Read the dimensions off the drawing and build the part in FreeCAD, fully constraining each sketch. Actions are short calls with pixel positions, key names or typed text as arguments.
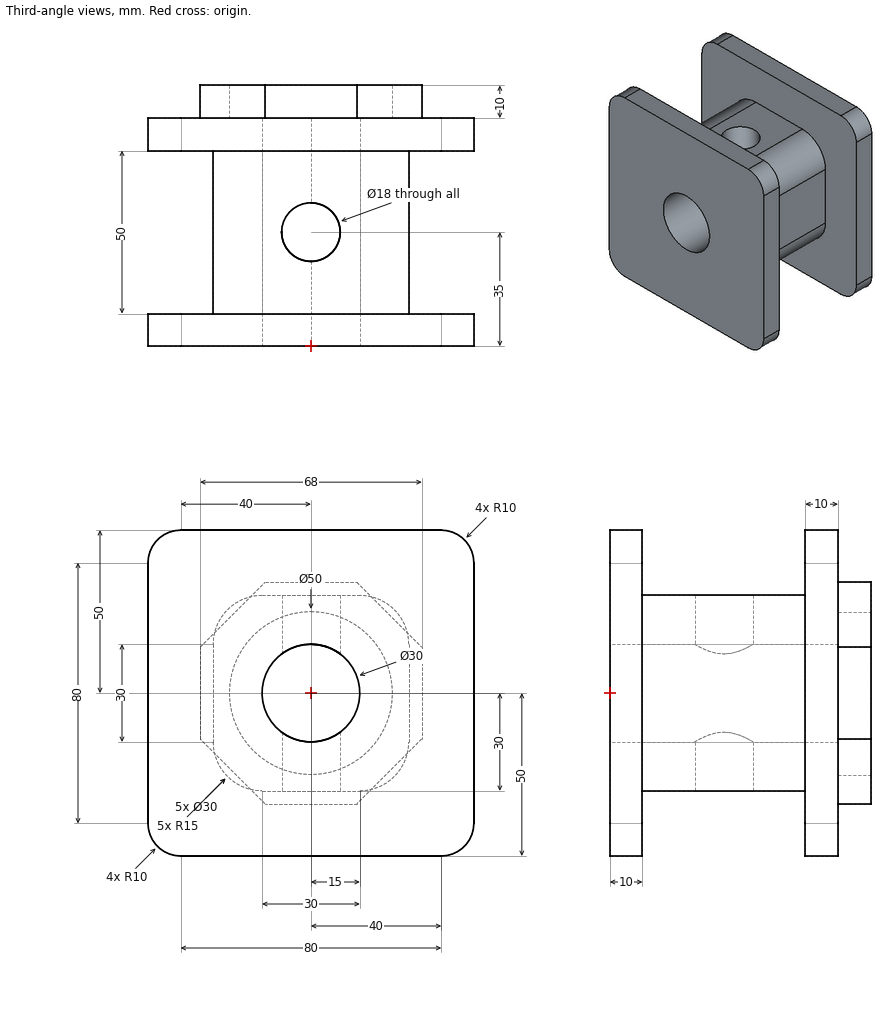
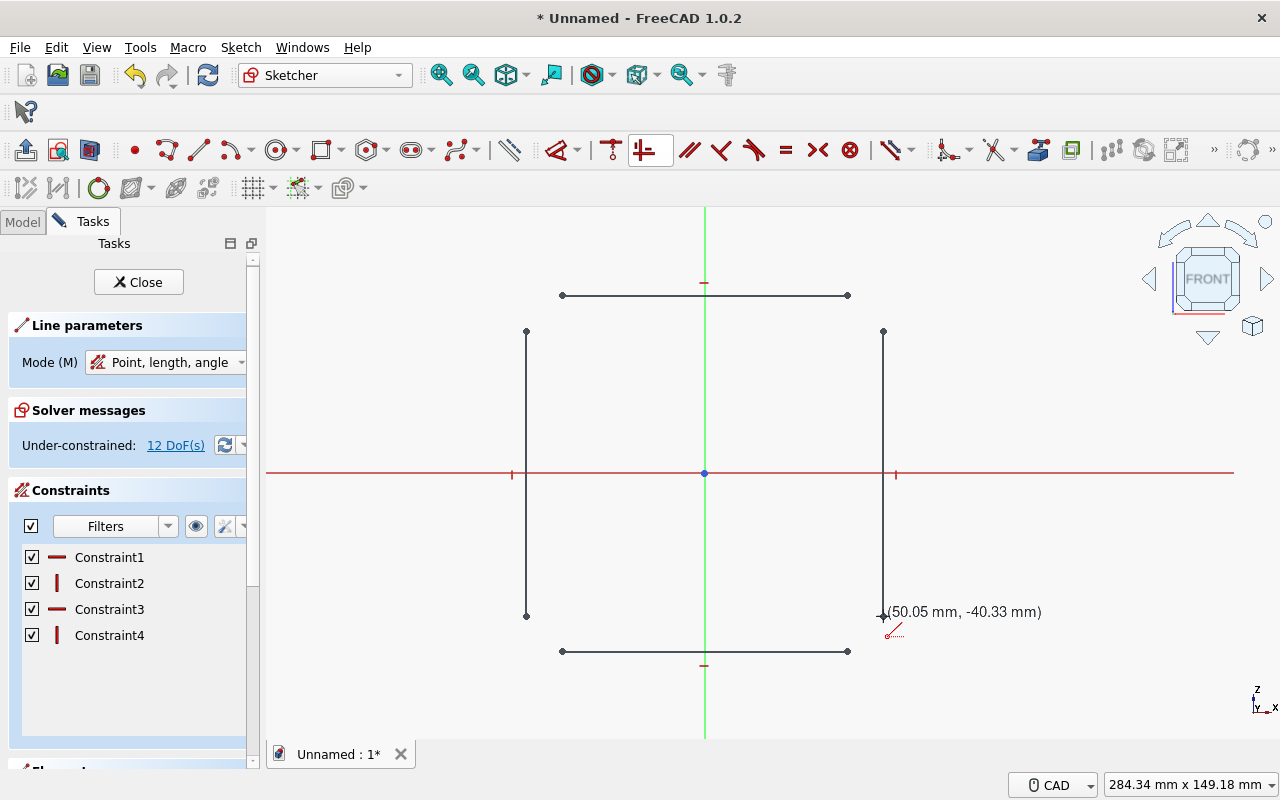
click(254, 150)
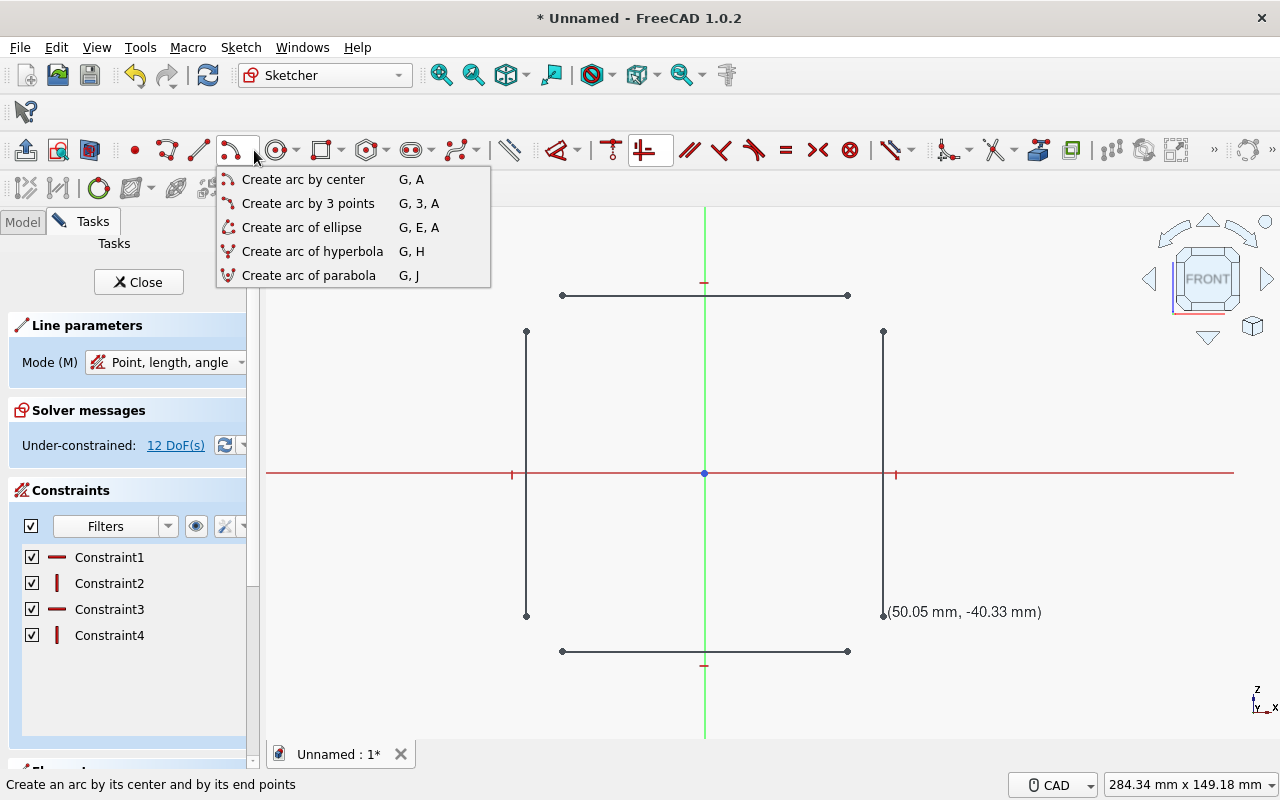
click(354, 203)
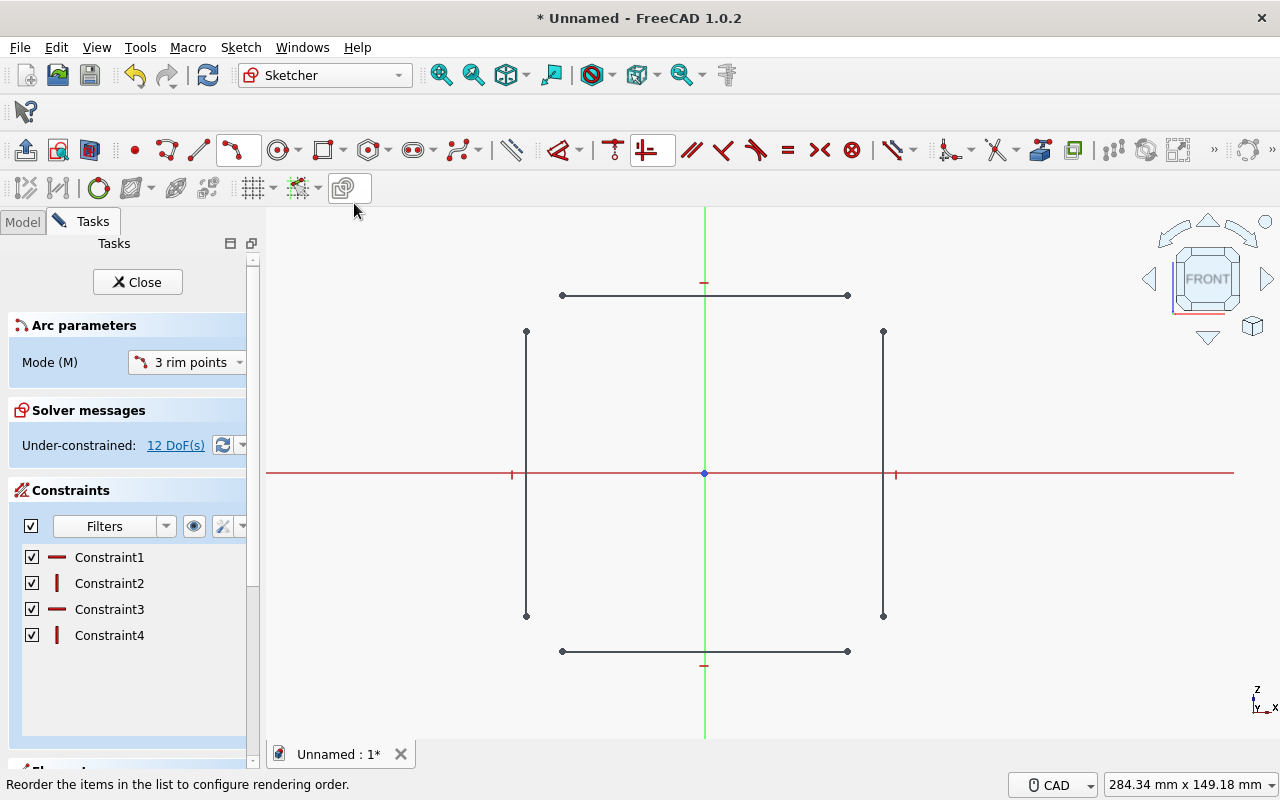
click(562, 652)
click(526, 617)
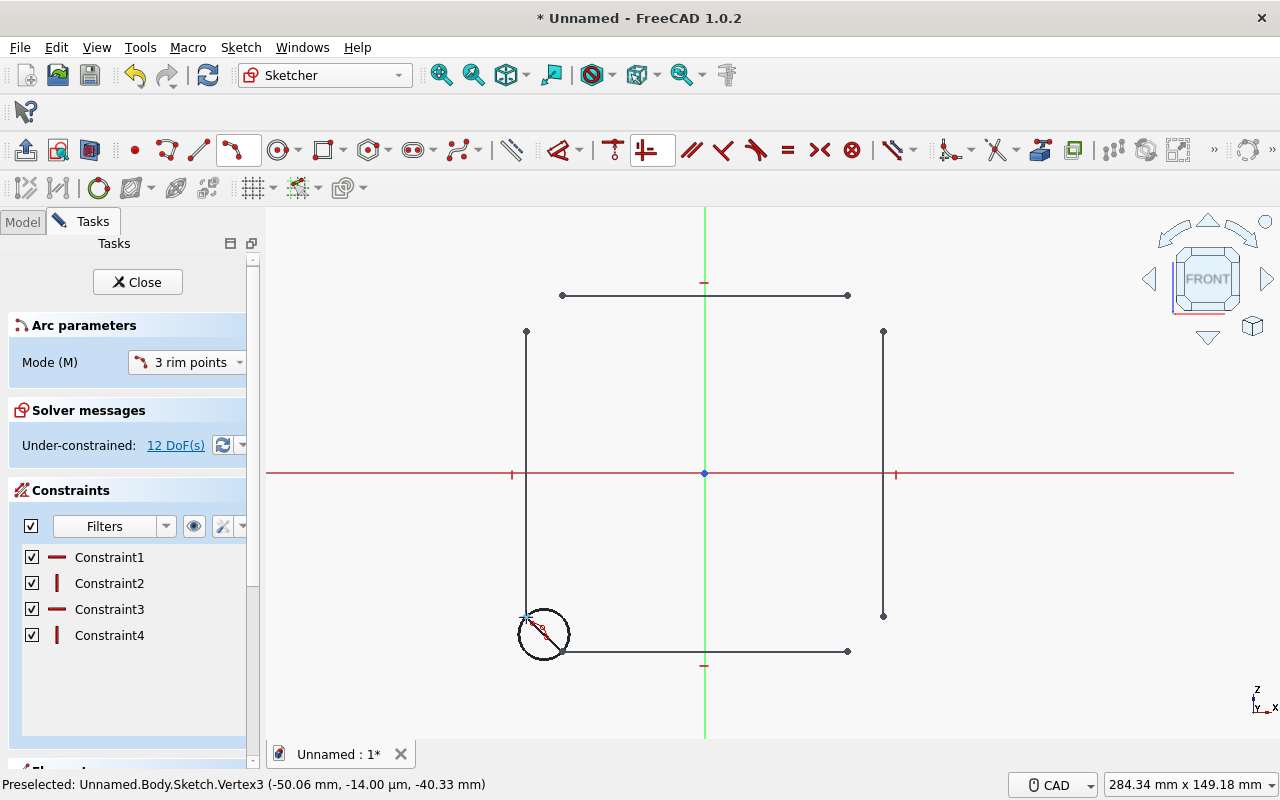
scroll(537, 641, up, 3)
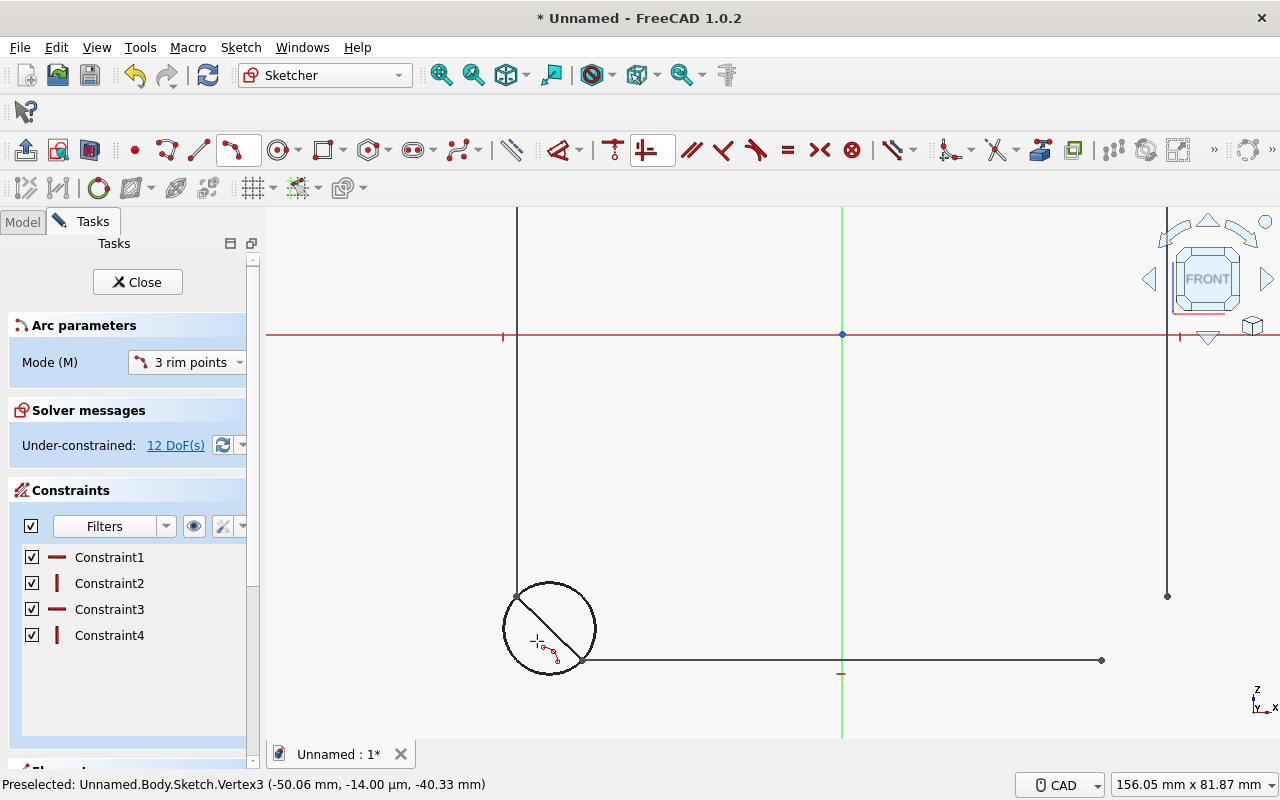
click(536, 640)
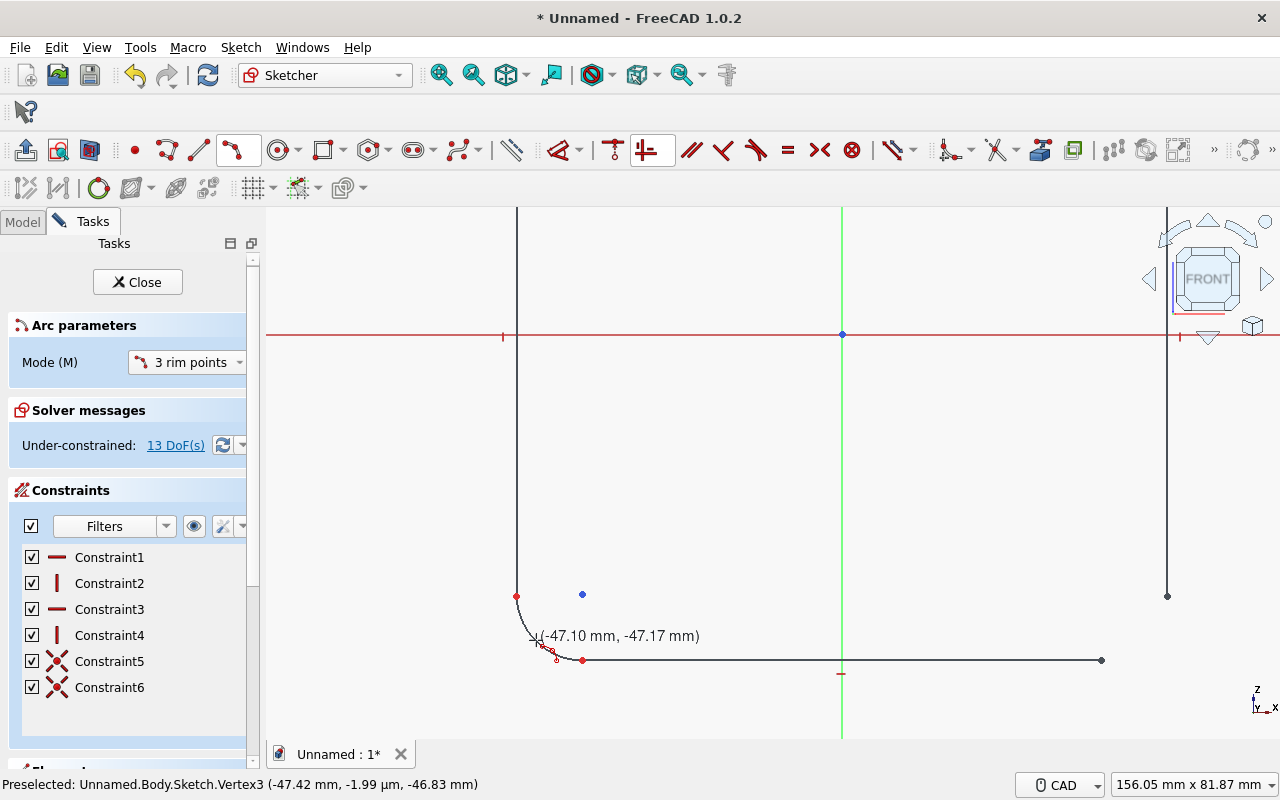
scroll(537, 641, down, 3)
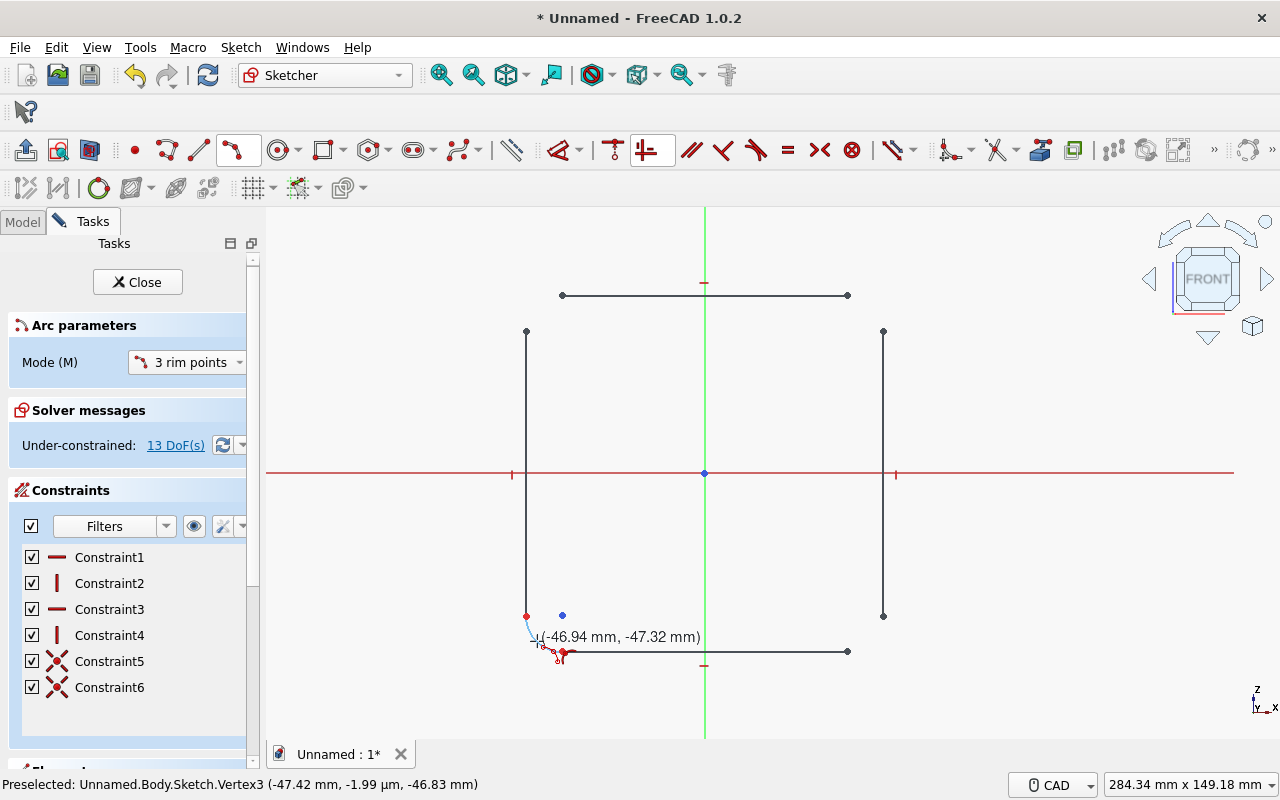
click(526, 332)
click(562, 296)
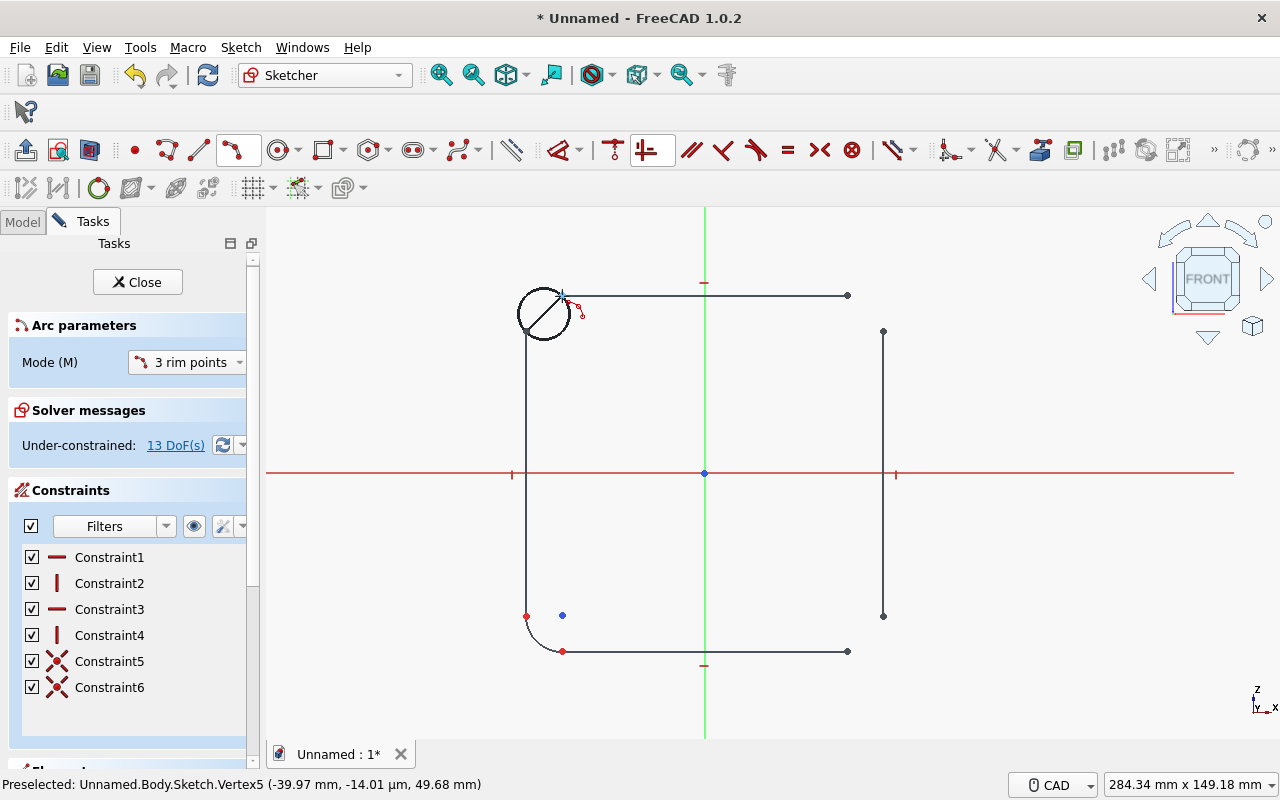
scroll(537, 305, up, 3)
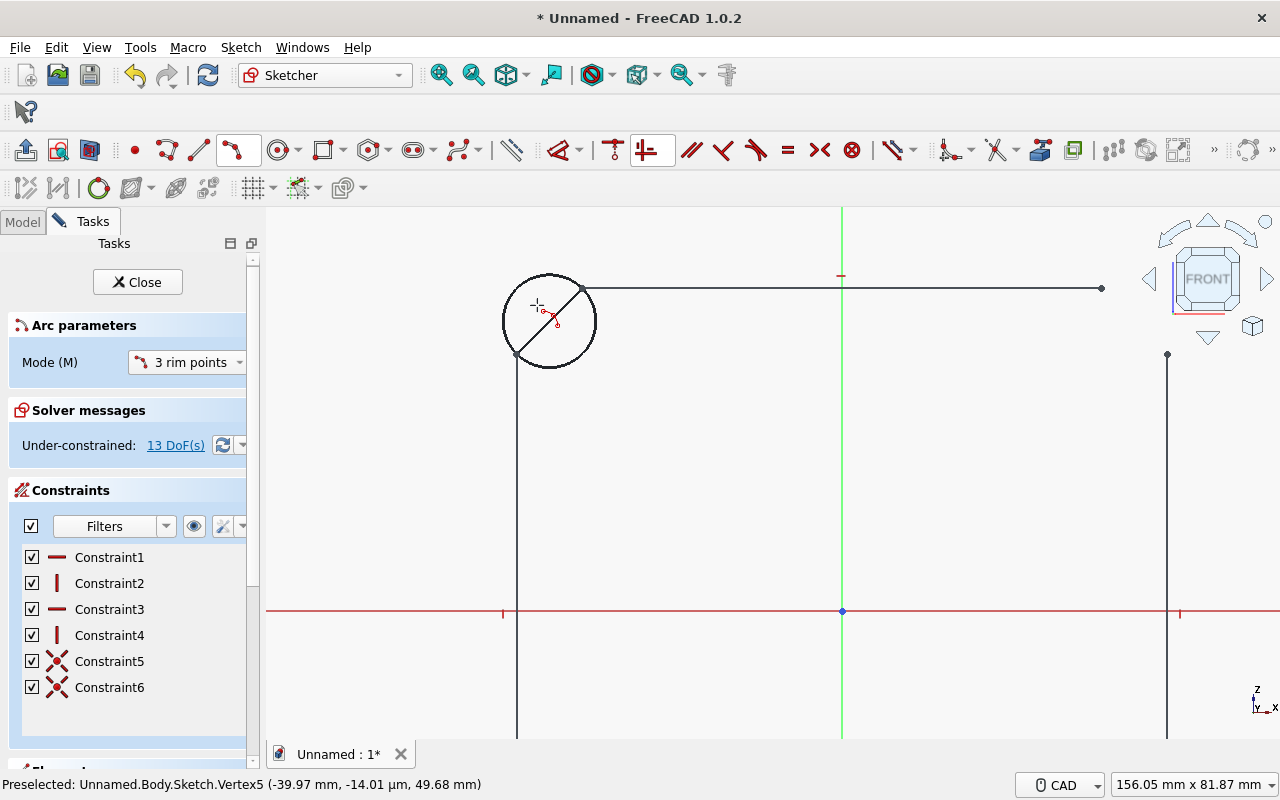
click(536, 305)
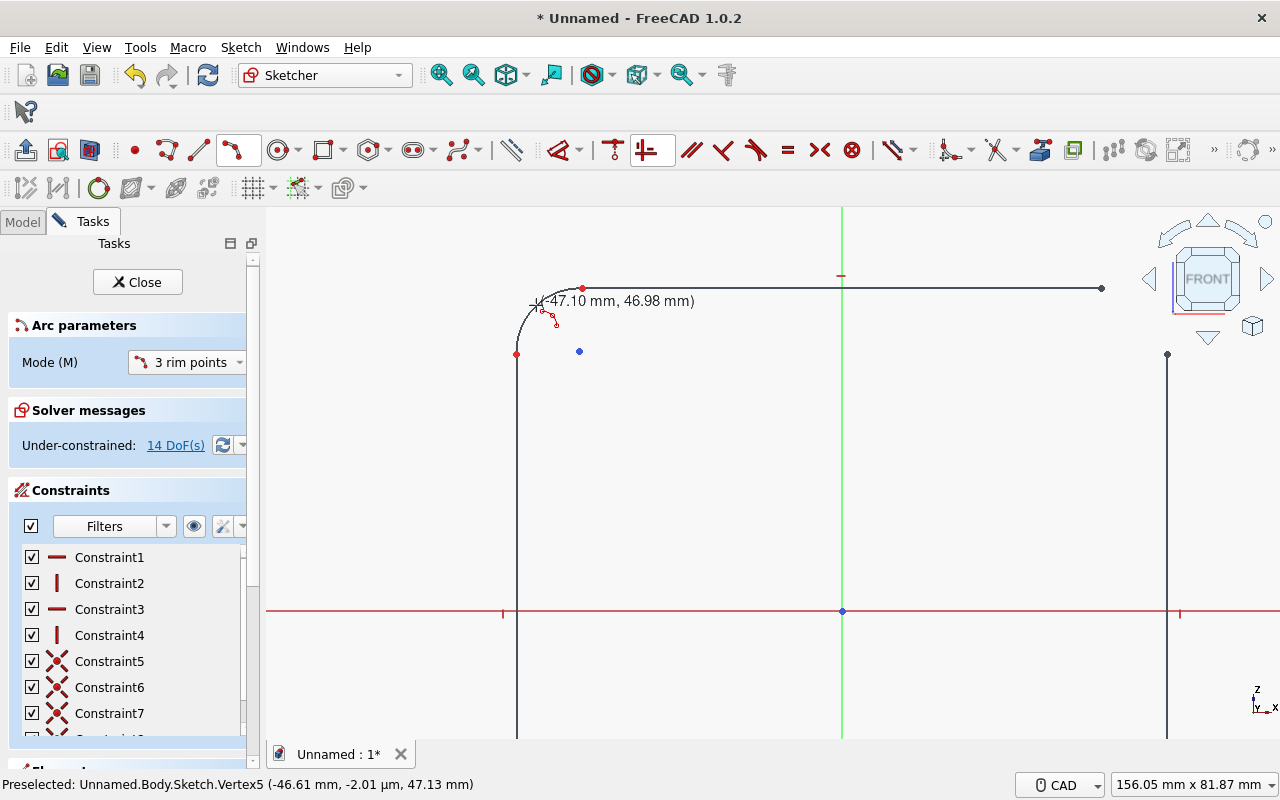
click(1102, 288)